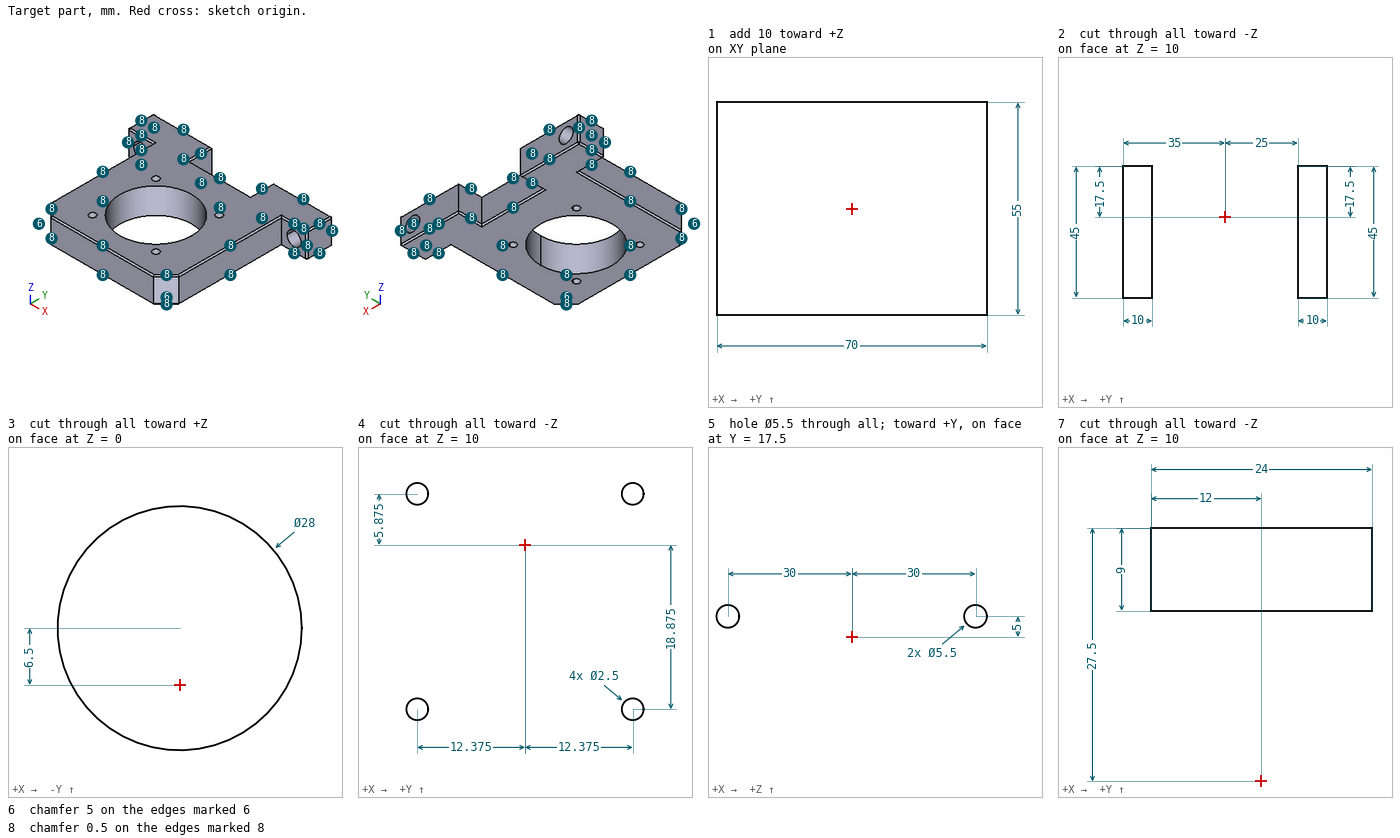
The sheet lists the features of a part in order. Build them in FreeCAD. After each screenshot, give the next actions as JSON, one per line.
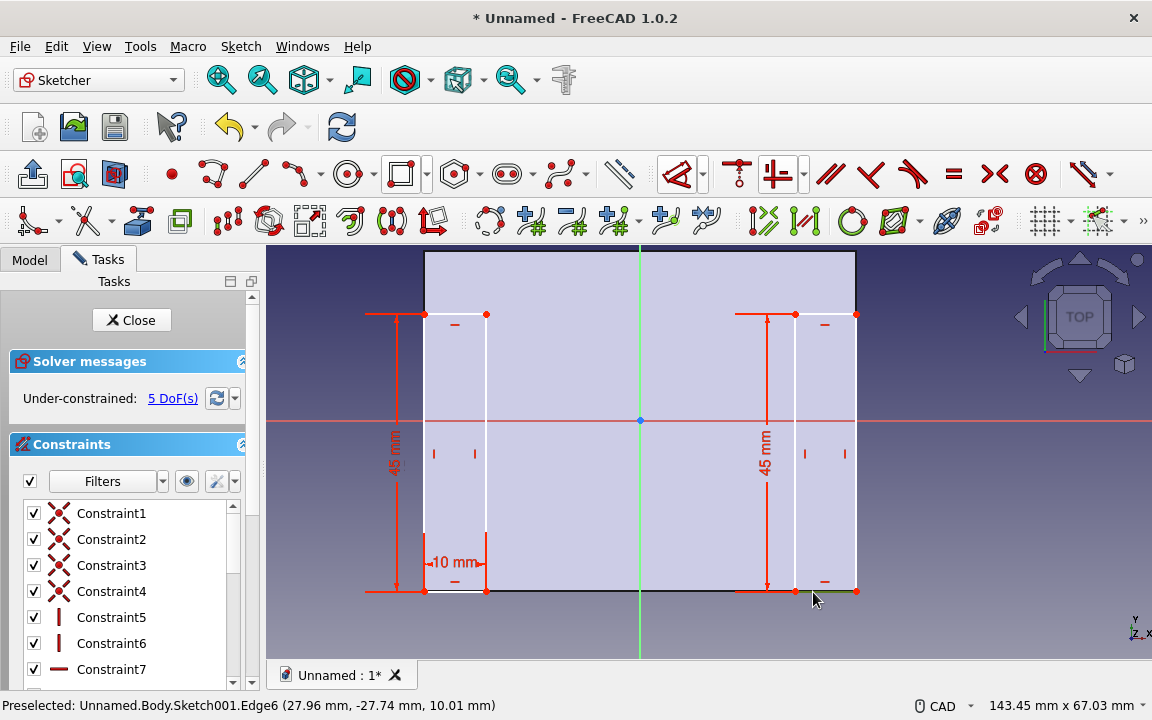
{"action": "key", "text": "l"}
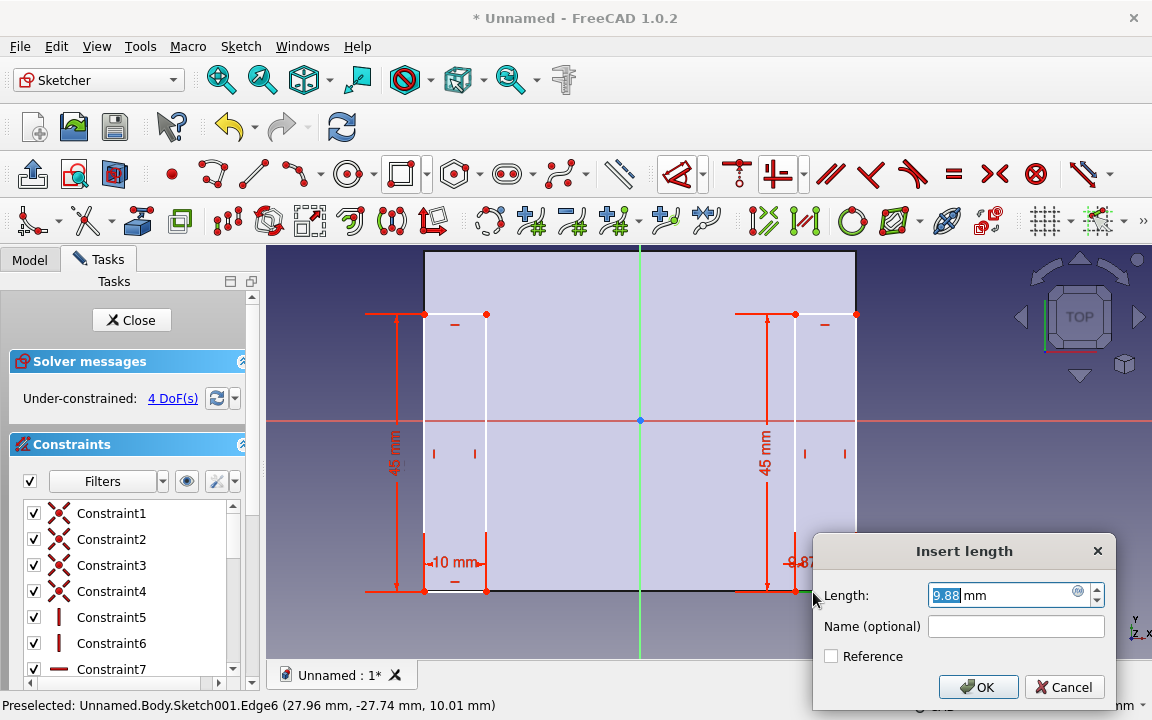
{"action": "type", "text": "10"}
{"action": "key", "text": "Return"}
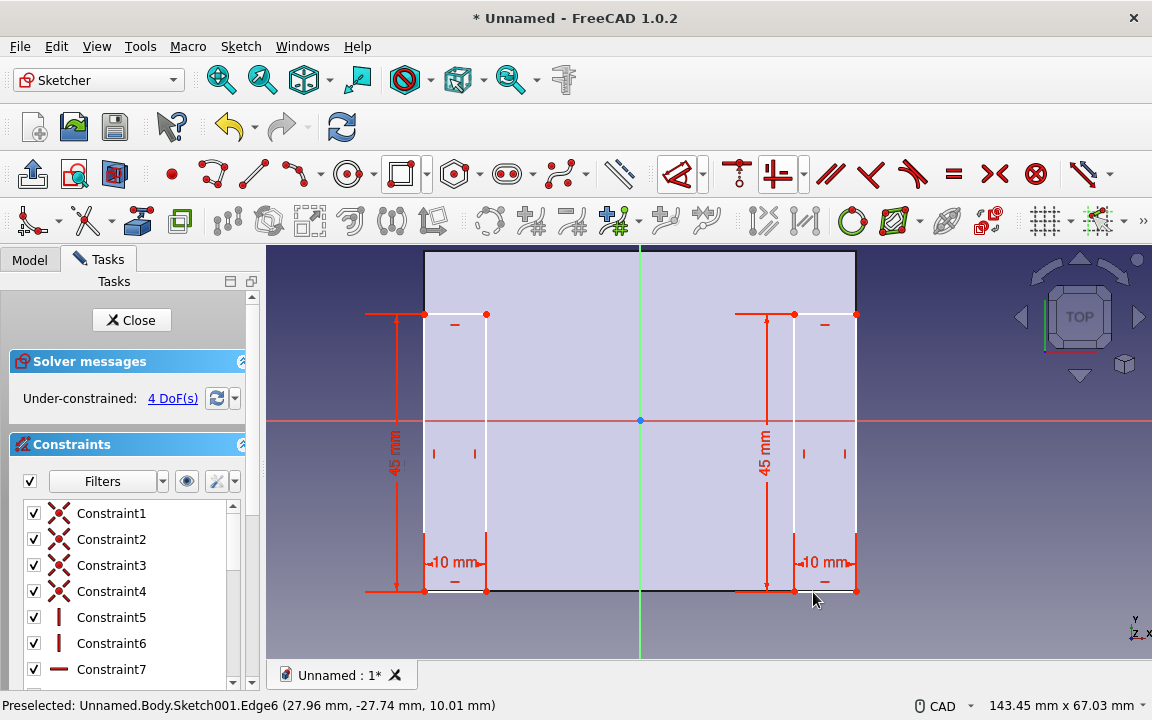
{"action": "left_click", "coordinate": [424, 314]}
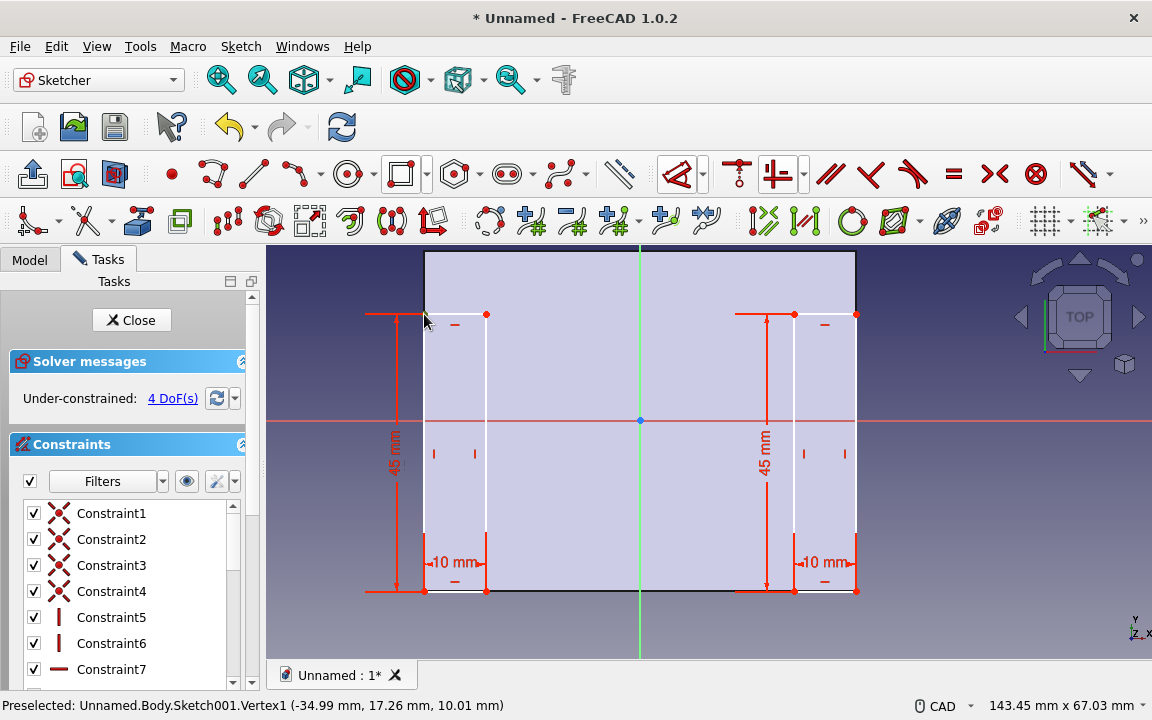
{"action": "left_click", "coordinate": [702, 174]}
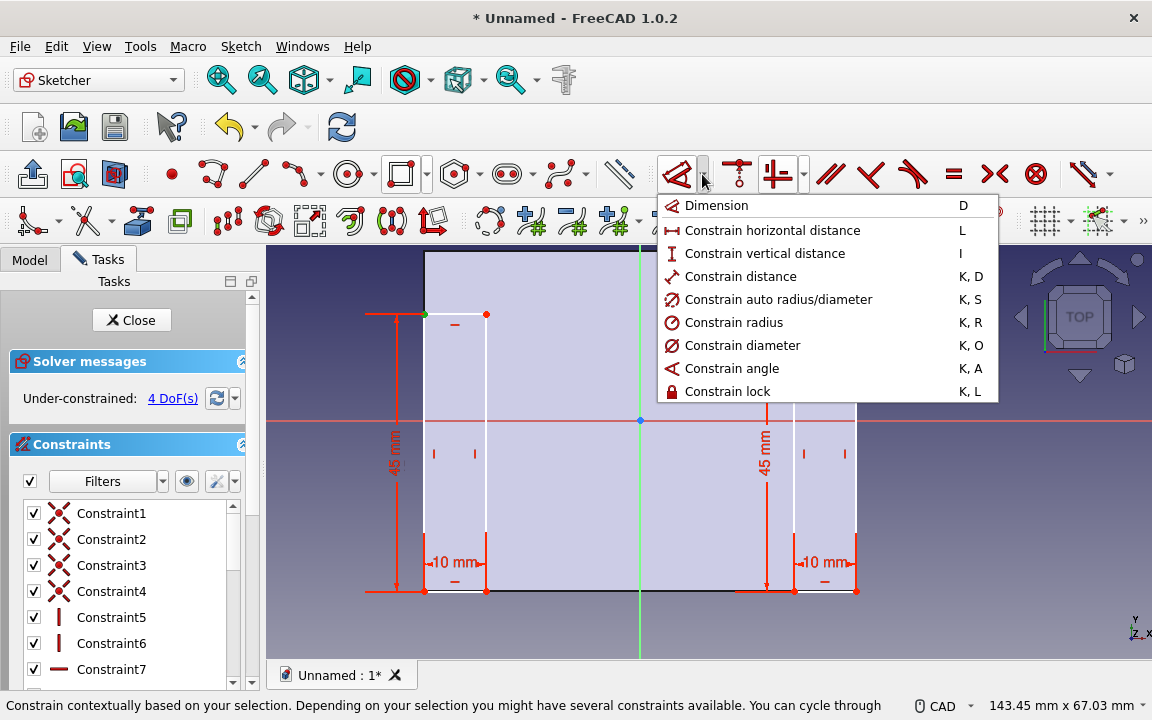
{"action": "left_click", "coordinate": [828, 230]}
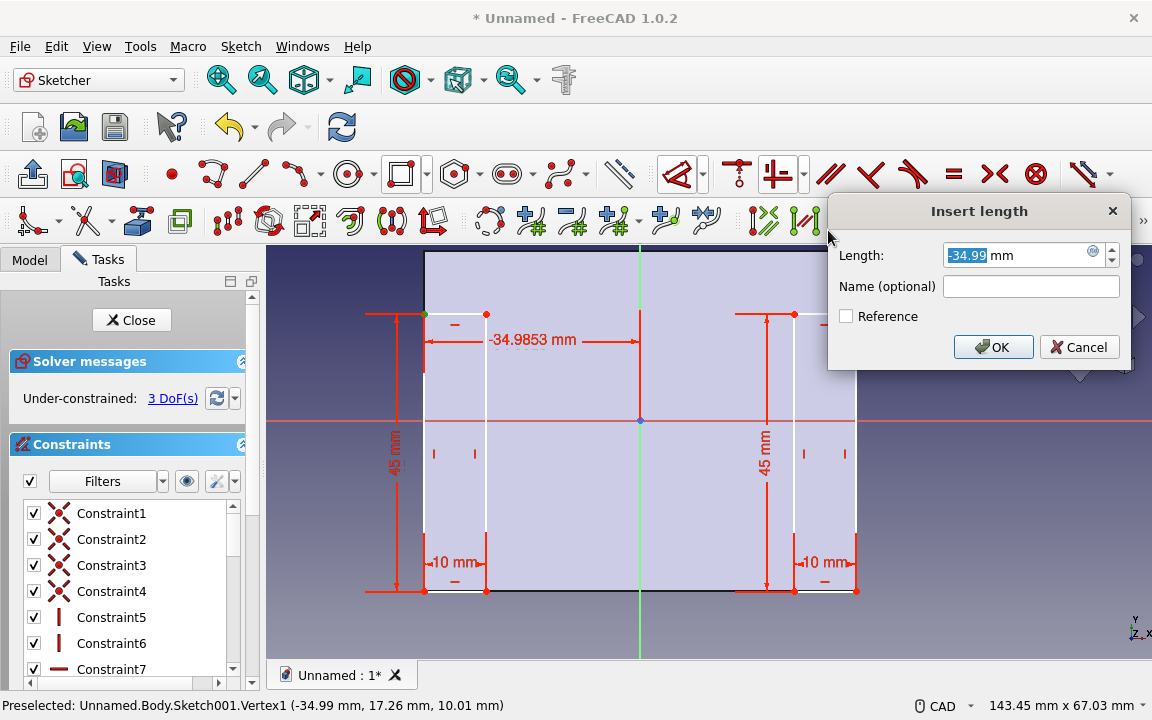
{"action": "type", "text": "-35"}
{"action": "key", "text": "Return"}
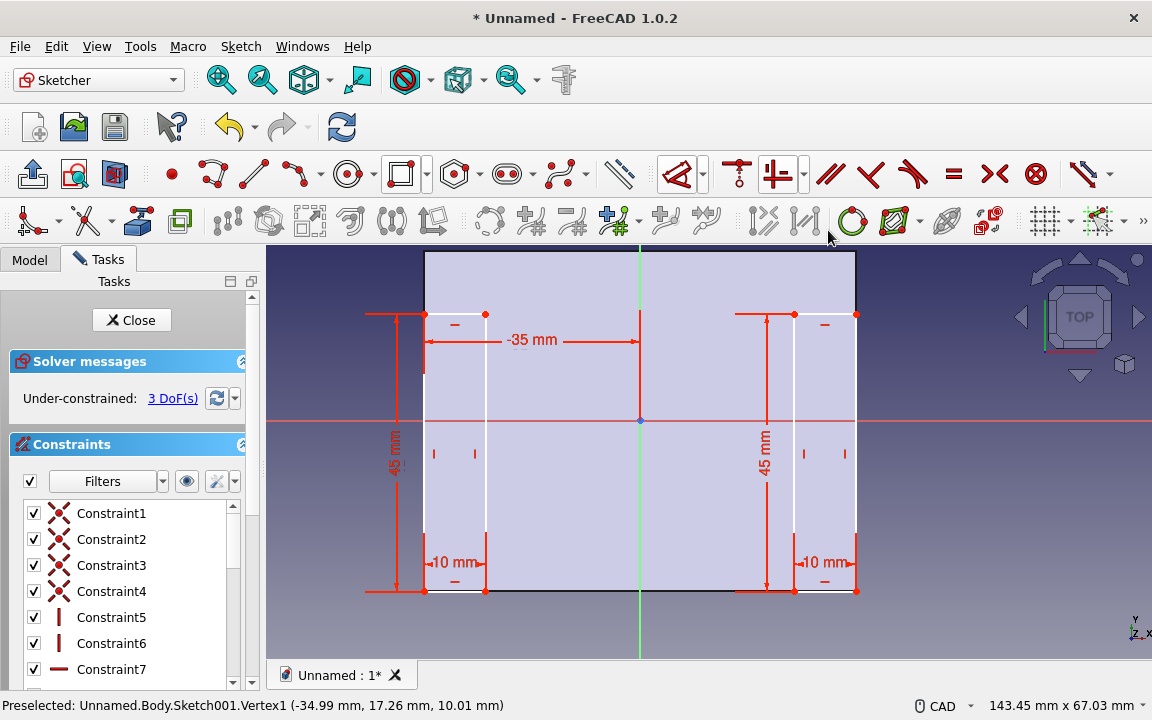
{"action": "left_click", "coordinate": [794, 314]}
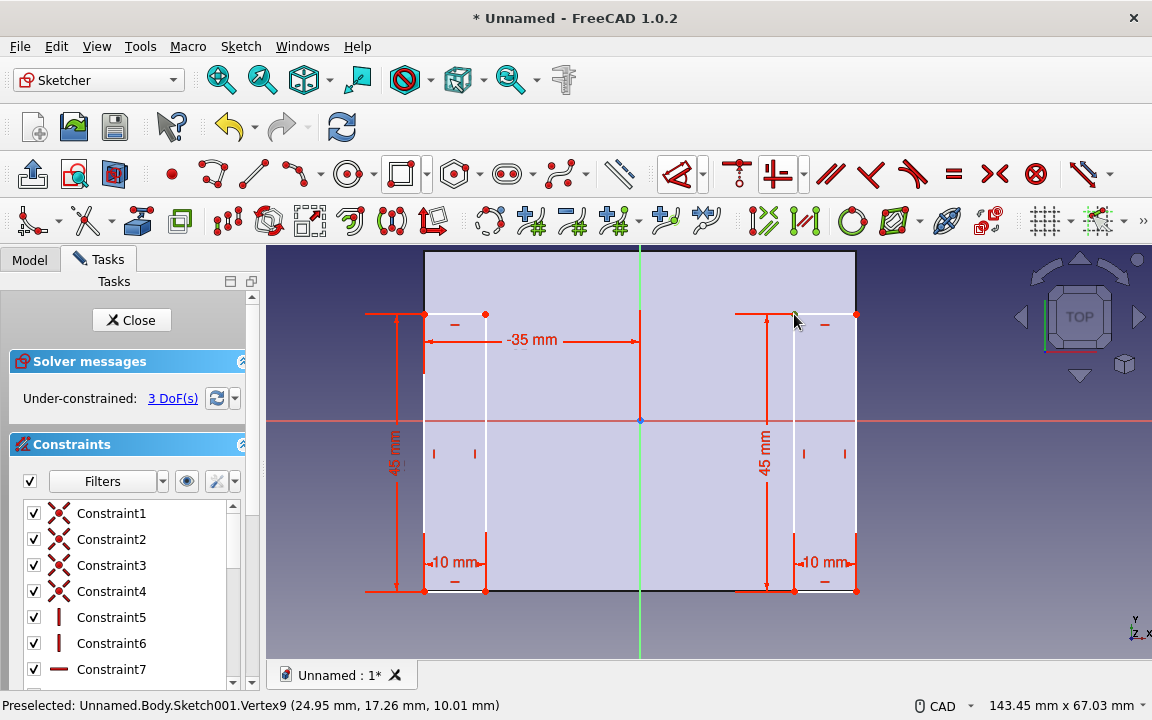
{"action": "key", "text": "l"}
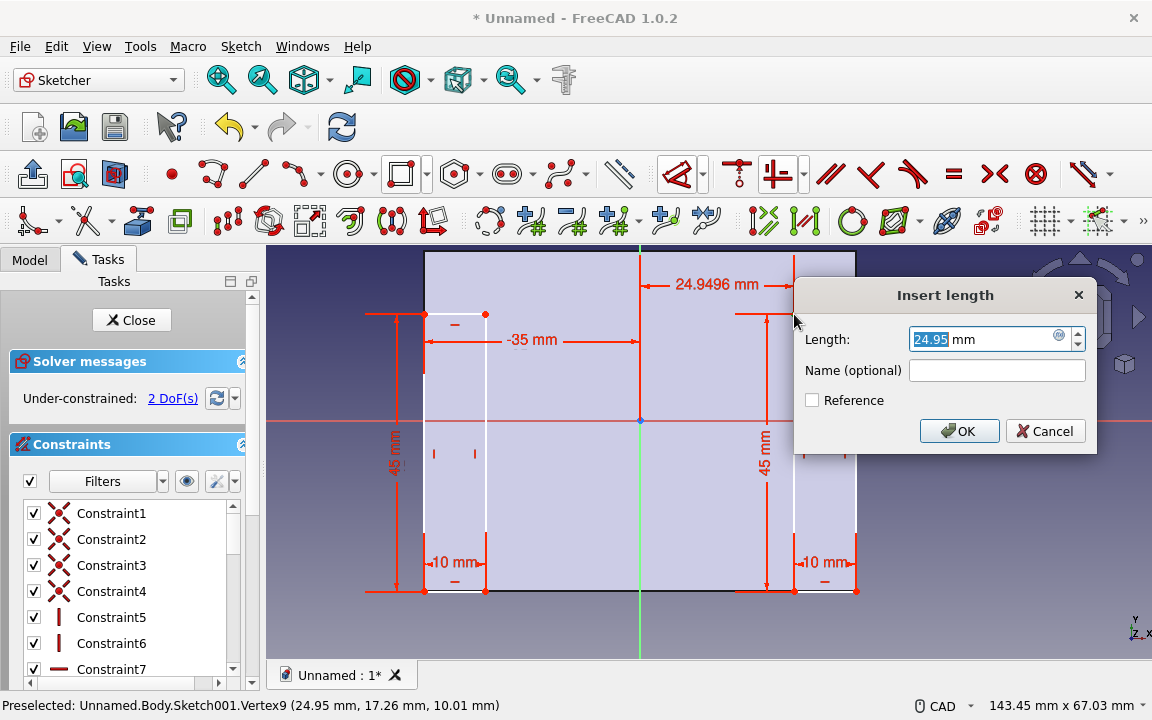
{"action": "type", "text": "25"}
{"action": "key", "text": "Return"}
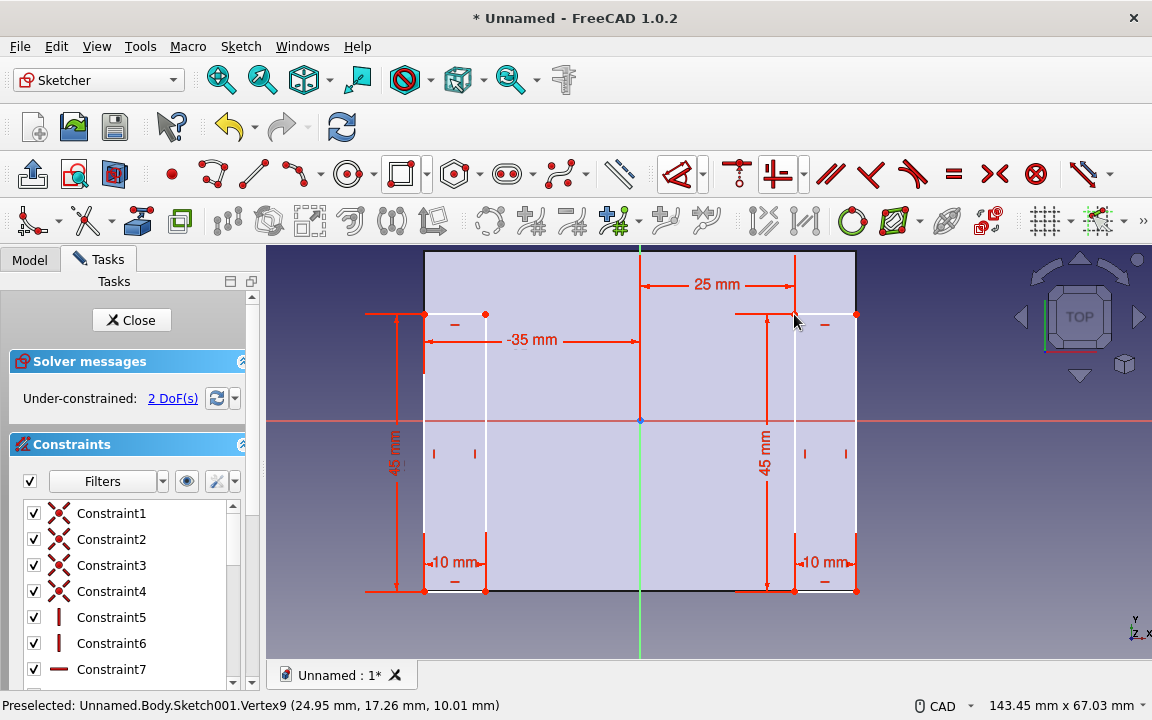
{"action": "left_click", "coordinate": [424, 314]}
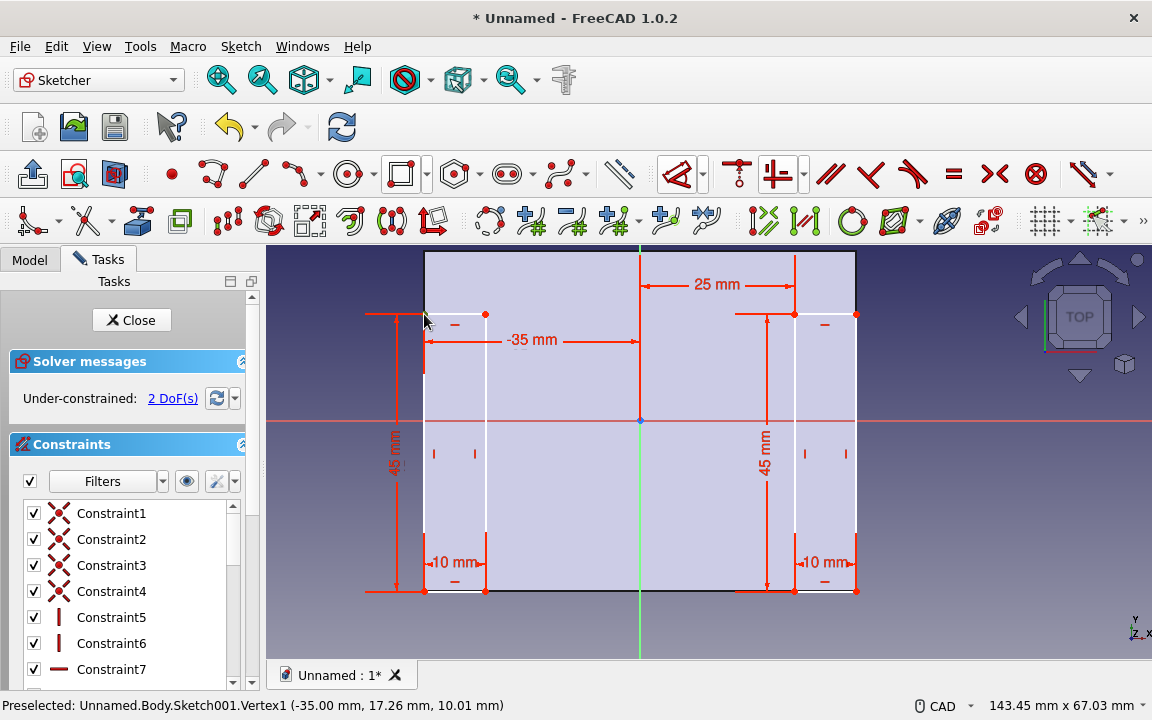
{"action": "left_click", "coordinate": [702, 174]}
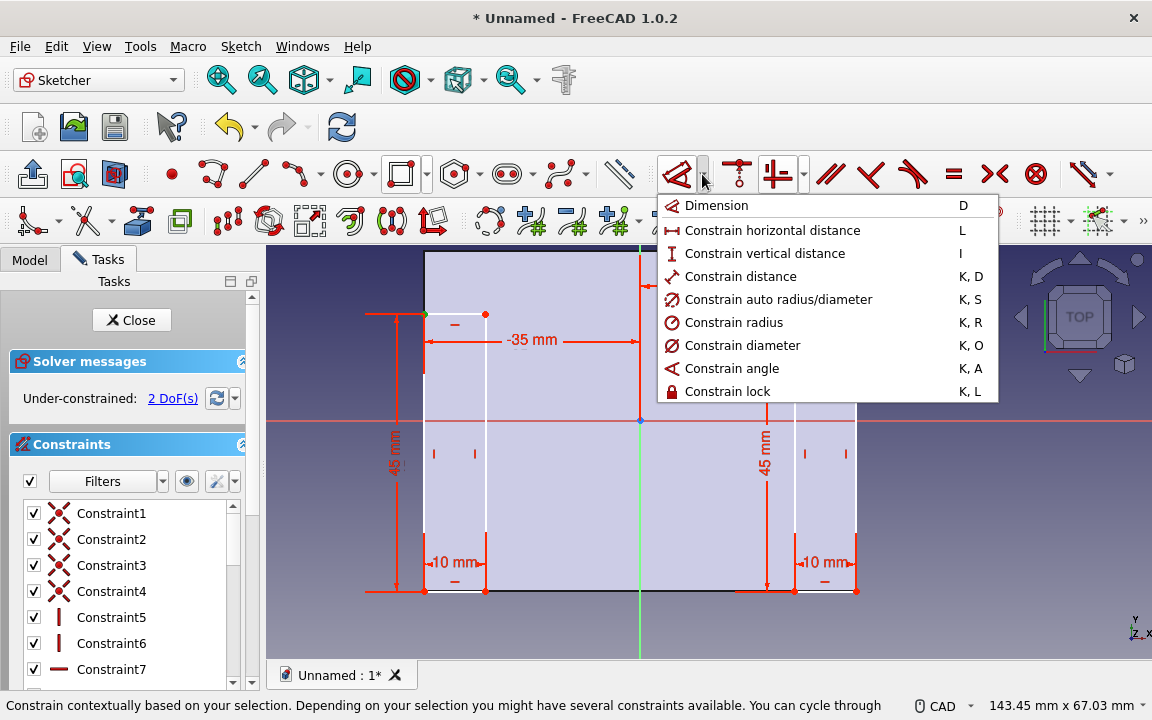
{"action": "left_click", "coordinate": [828, 254]}